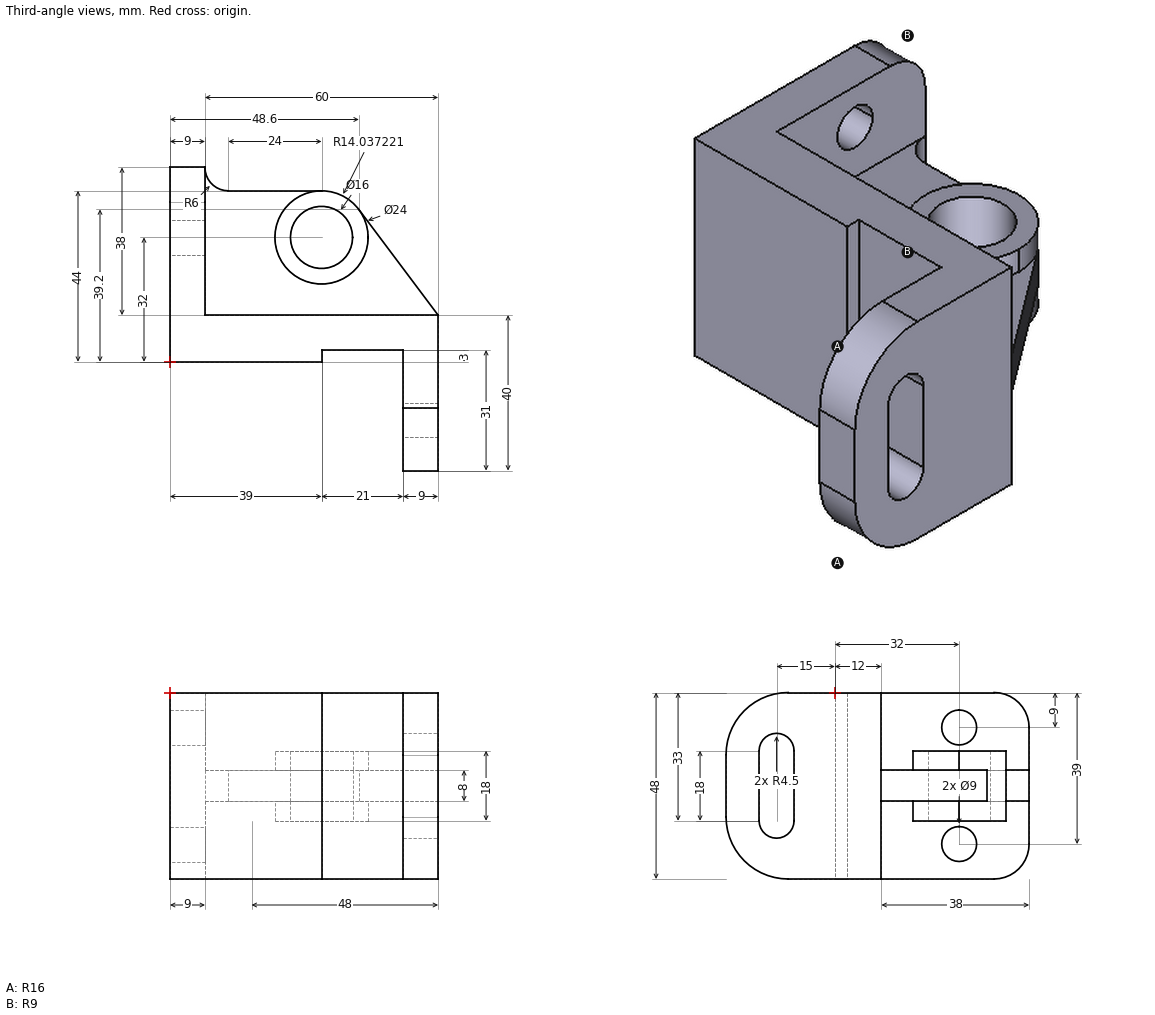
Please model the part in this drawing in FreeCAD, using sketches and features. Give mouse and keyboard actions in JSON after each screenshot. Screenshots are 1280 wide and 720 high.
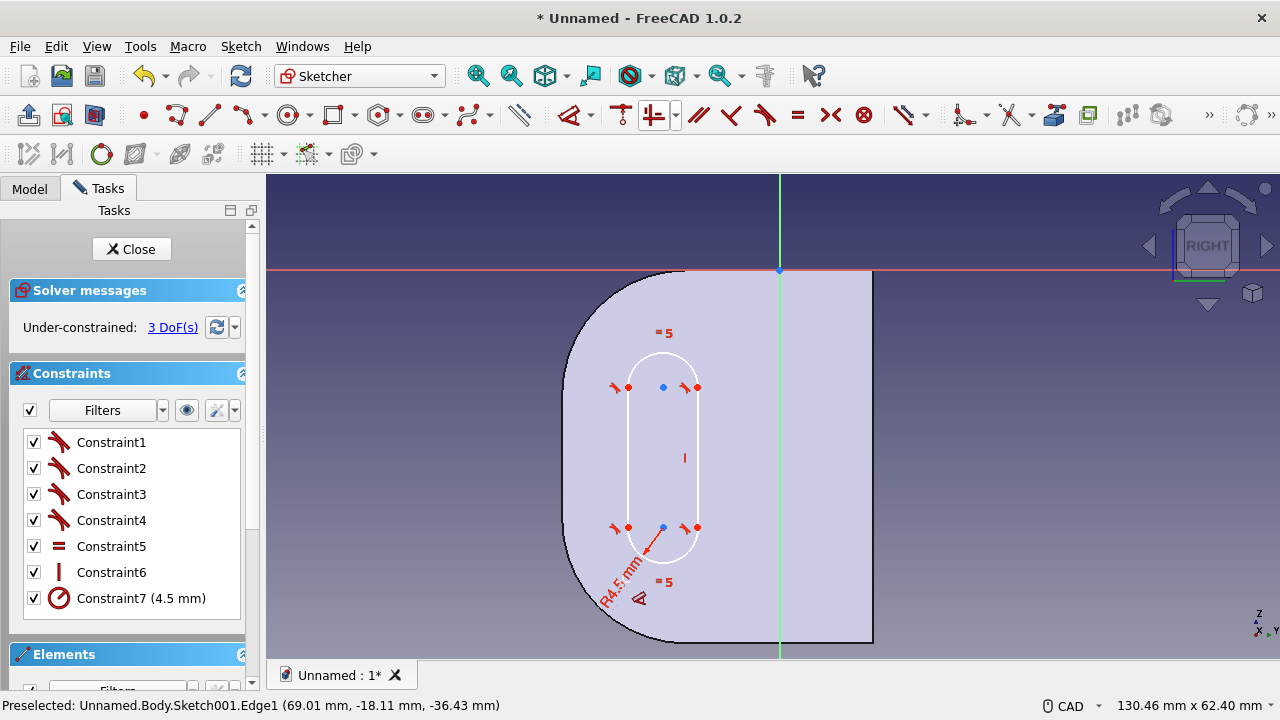
{"action": "left_click", "coordinate": [628, 486]}
{"action": "left_click", "coordinate": [594, 458]}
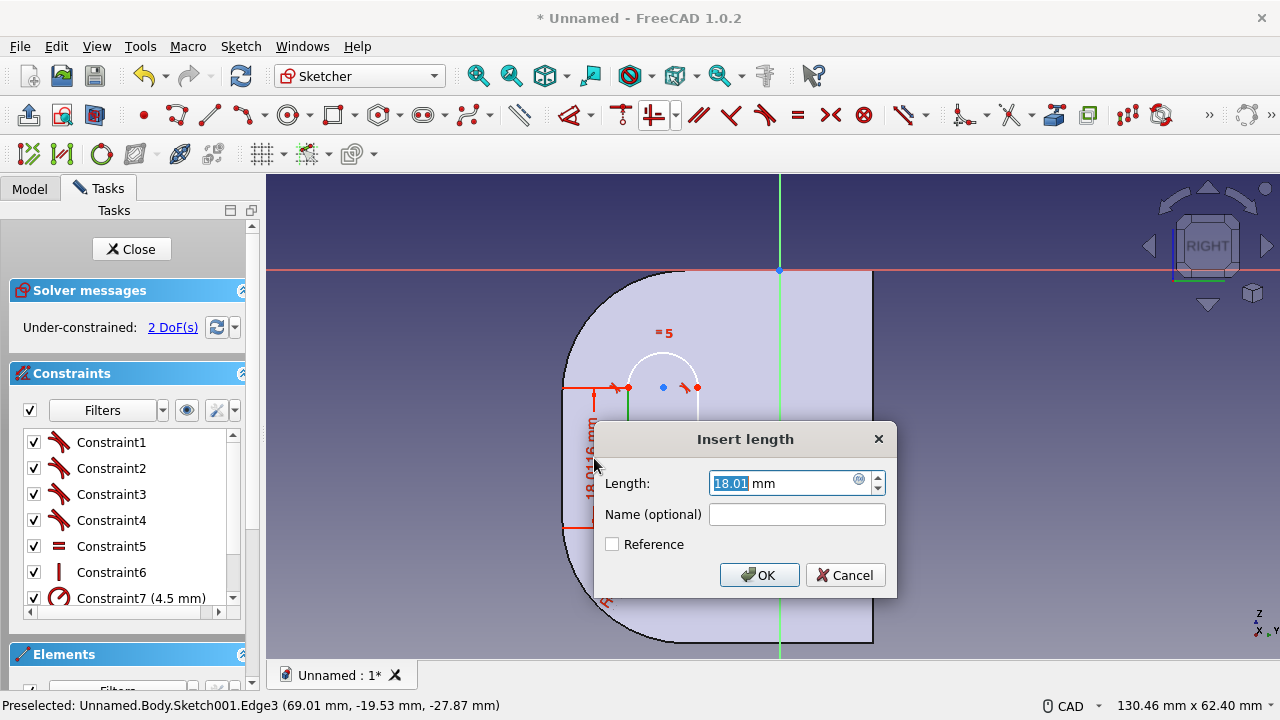
{"action": "type", "text": "18"}
{"action": "key", "text": "Return"}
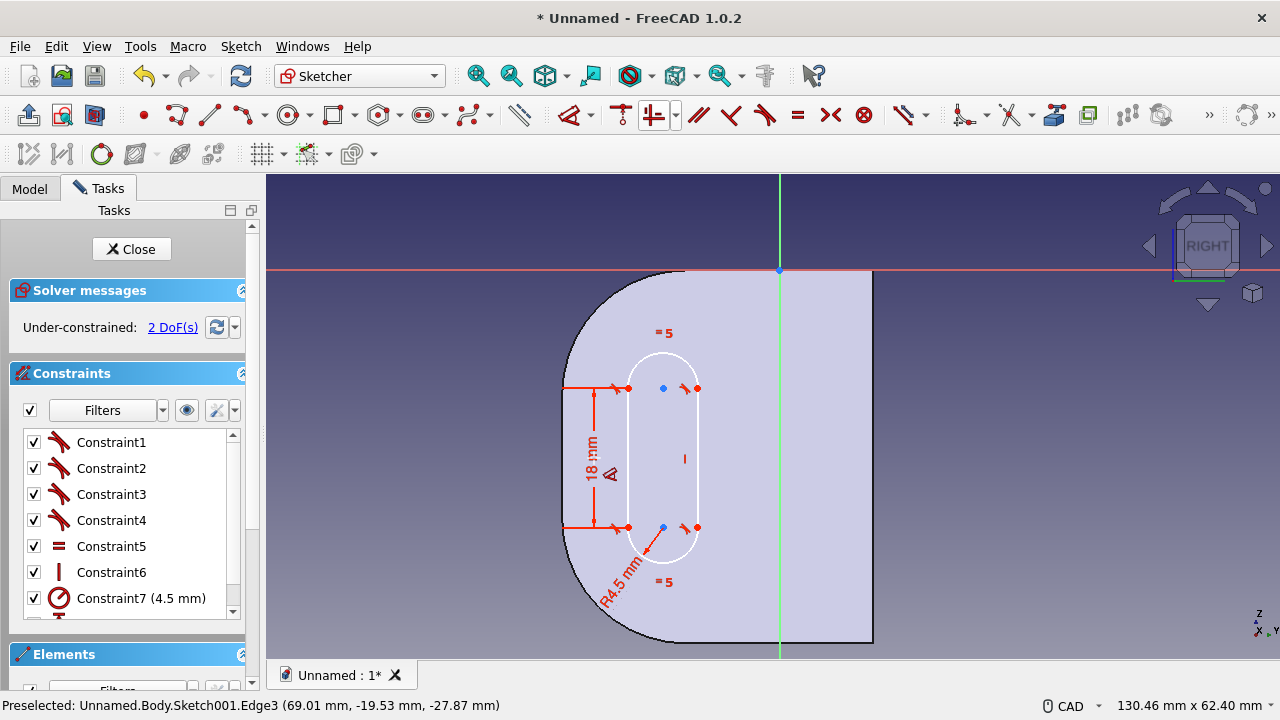
{"action": "left_click", "coordinate": [628, 528]}
{"action": "left_click", "coordinate": [594, 399]}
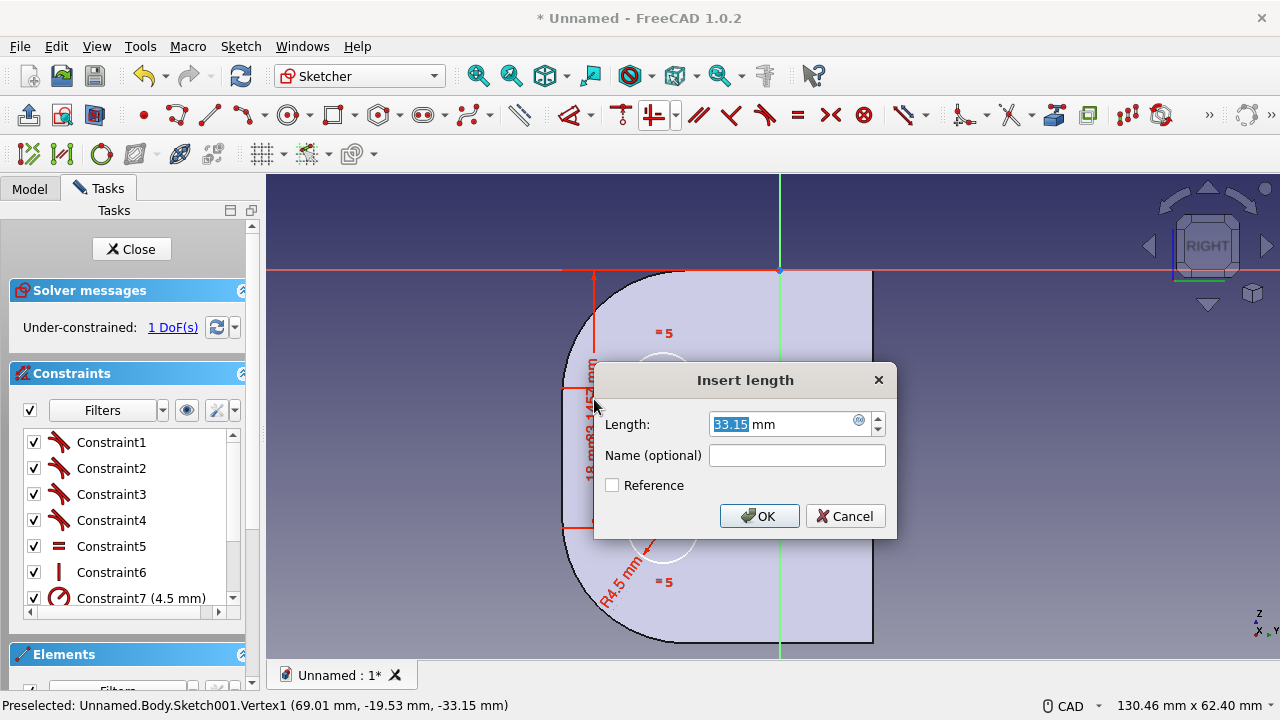
{"action": "type", "text": "33"}
{"action": "key", "text": "Return"}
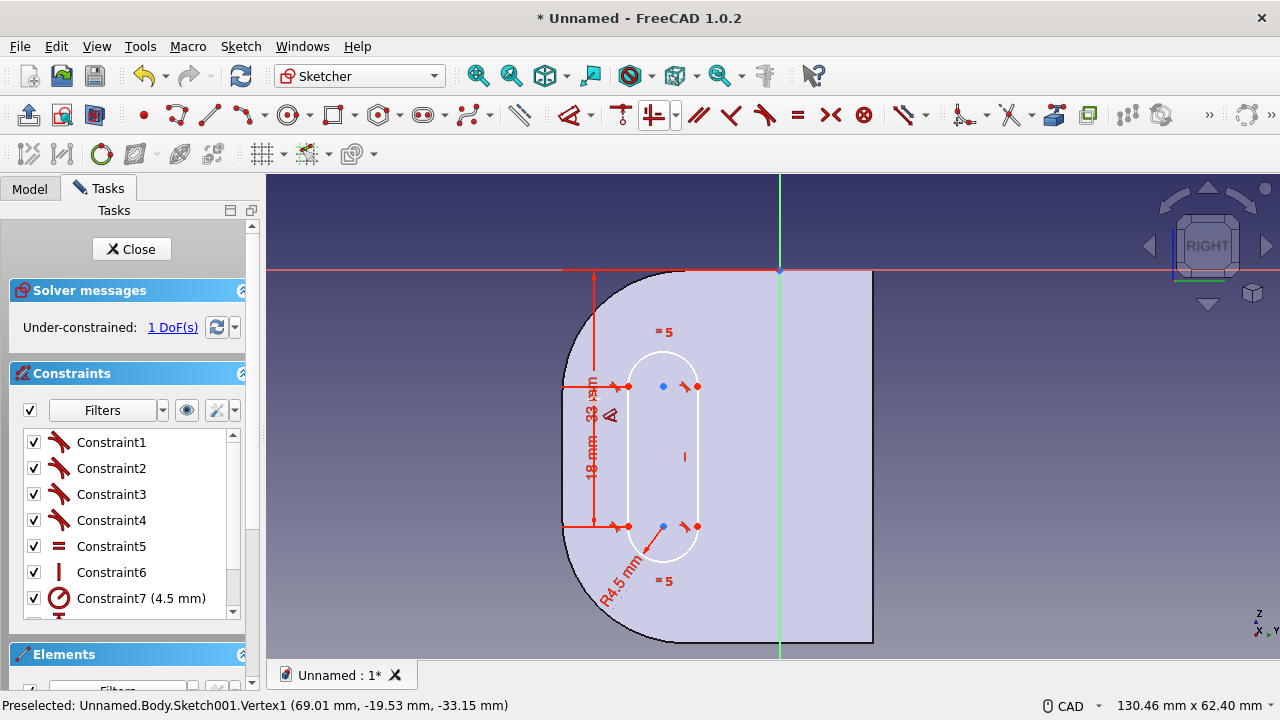
{"action": "left_click", "coordinate": [663, 527]}
{"action": "left_click", "coordinate": [721, 236]}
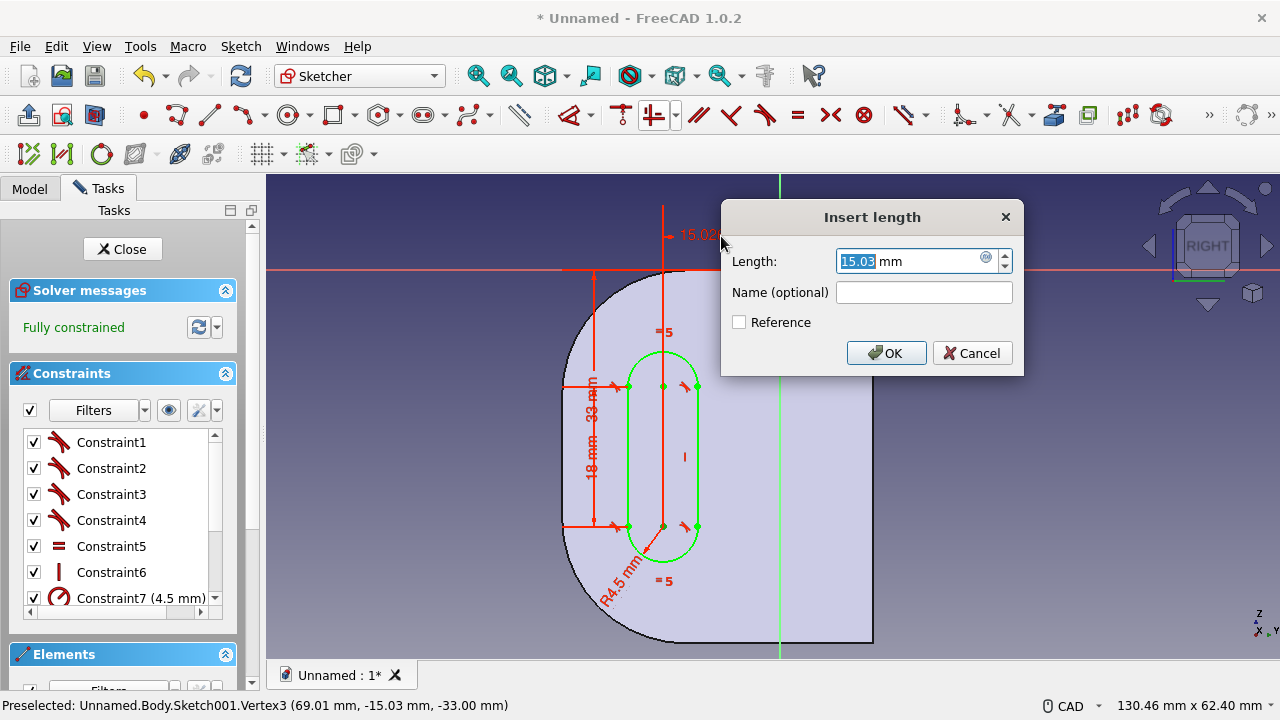
{"action": "type", "text": "15"}
{"action": "key", "text": "Return"}
{"action": "key", "text": "Escape"}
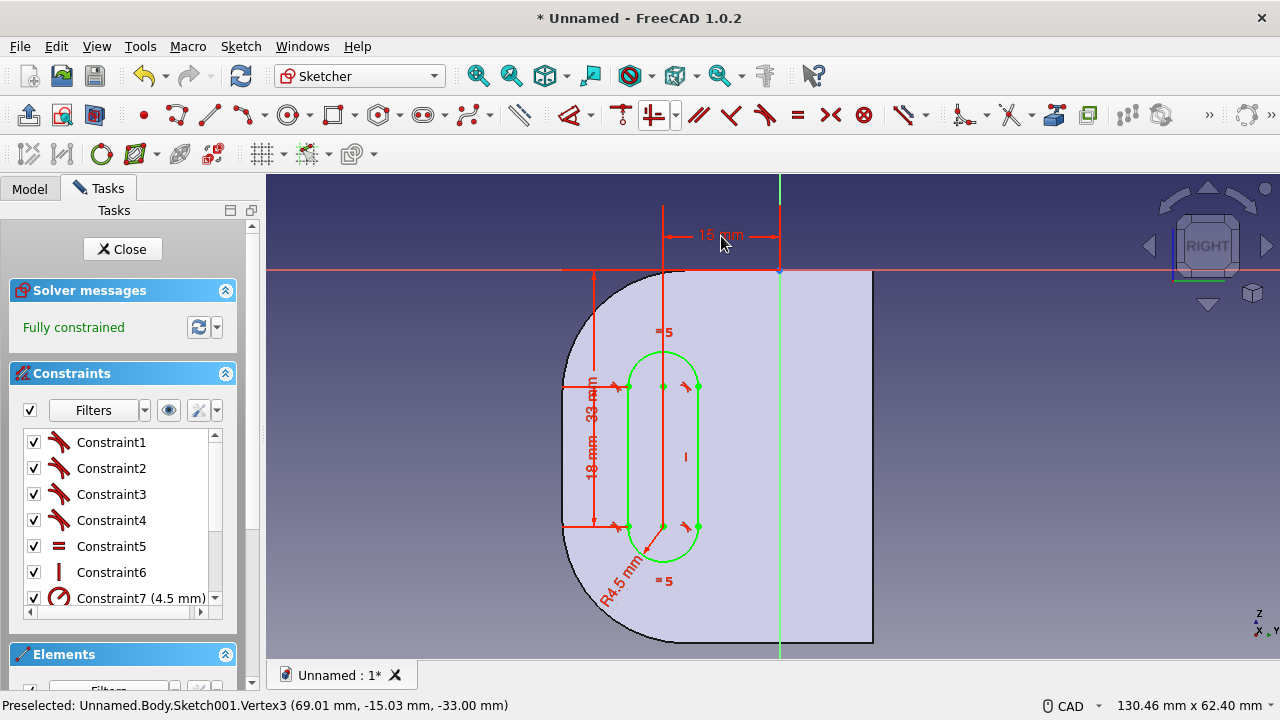
{"action": "left_click", "coordinate": [123, 249]}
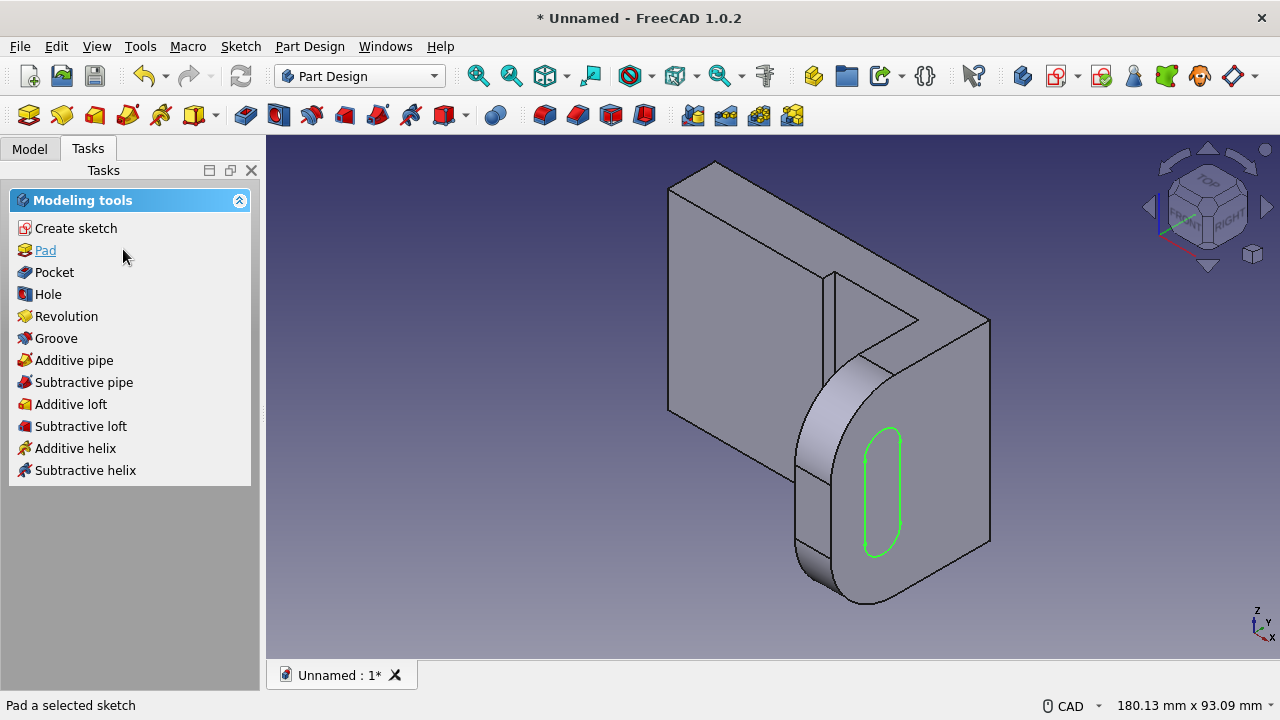
{"action": "left_click", "coordinate": [246, 116]}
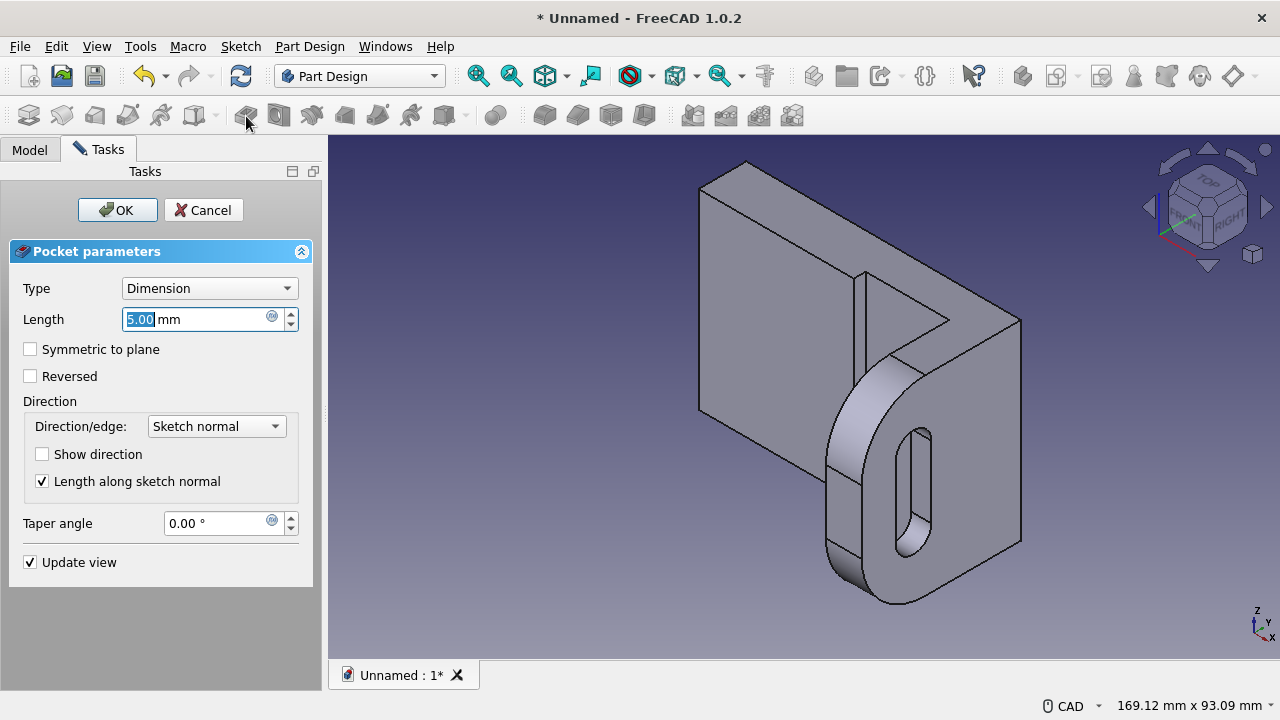
{"action": "type", "text": "48"}
{"action": "key", "text": "Tab"}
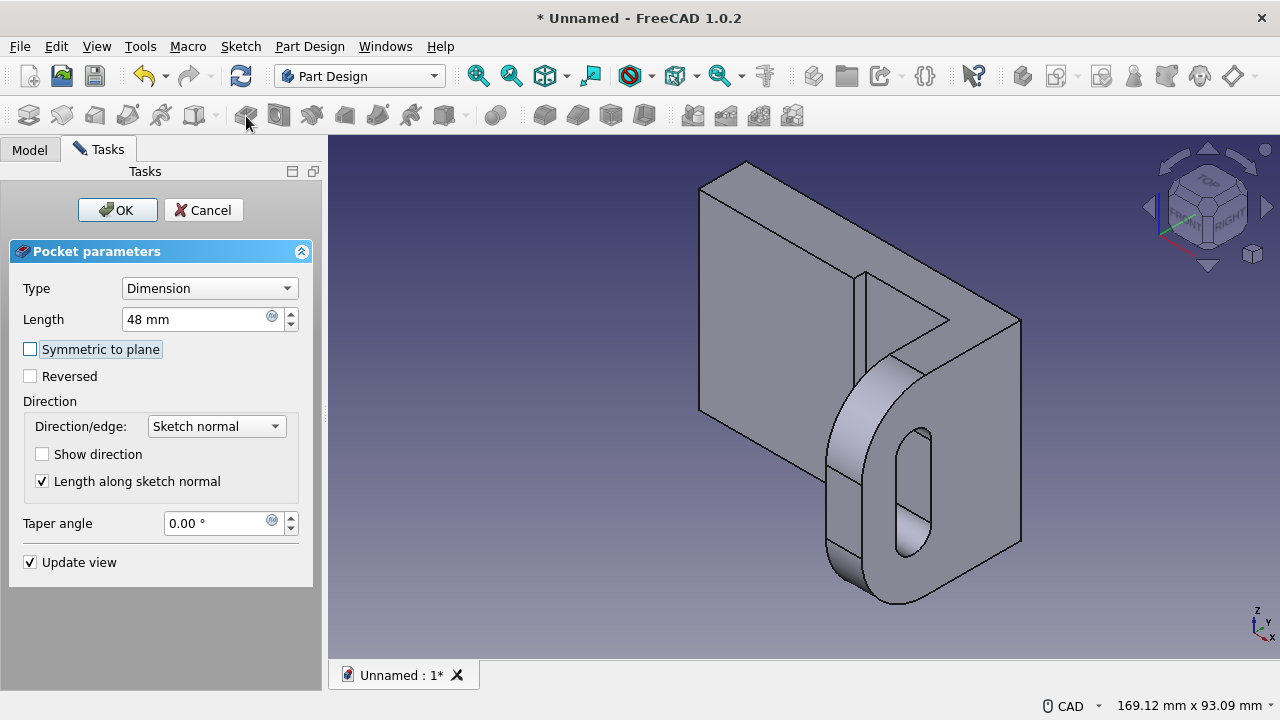
{"action": "left_click", "coordinate": [118, 210]}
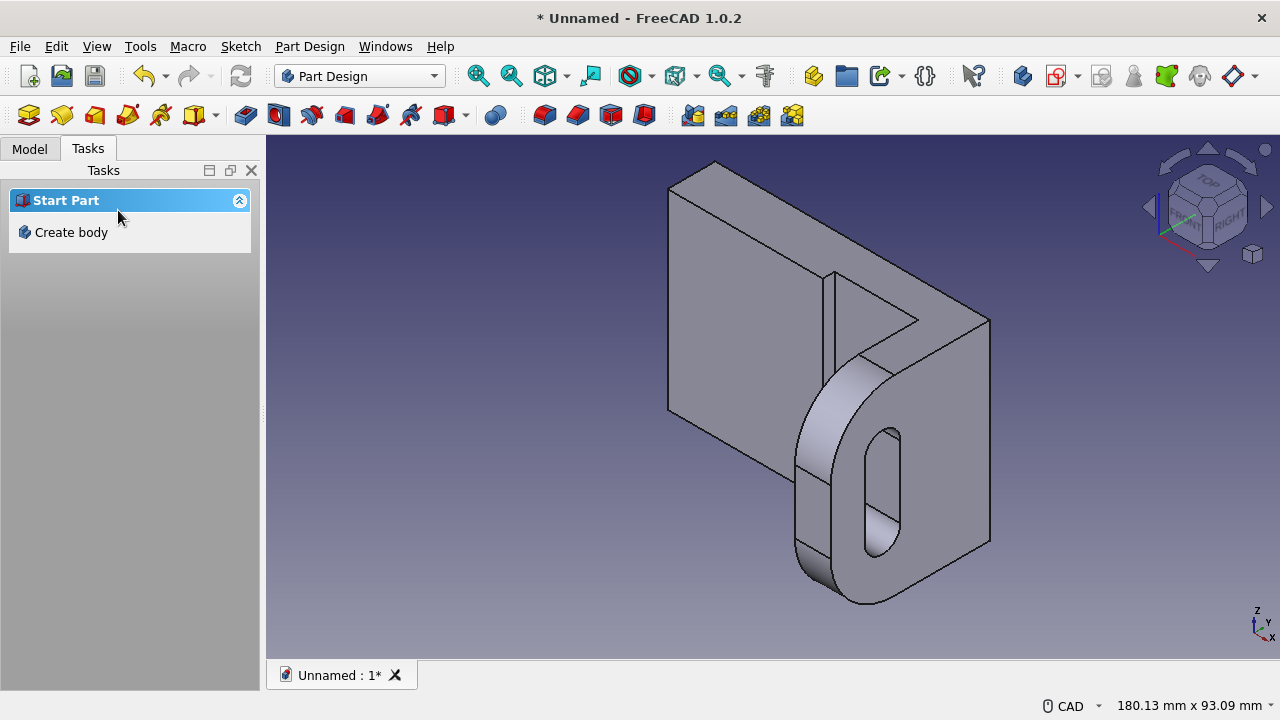
{"action": "left_click", "coordinate": [1056, 76]}